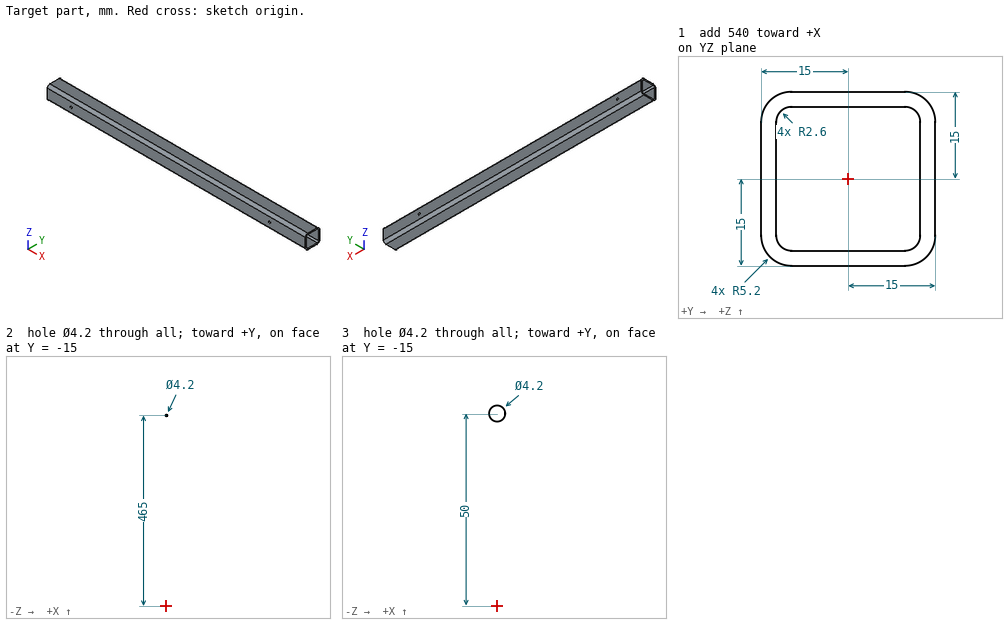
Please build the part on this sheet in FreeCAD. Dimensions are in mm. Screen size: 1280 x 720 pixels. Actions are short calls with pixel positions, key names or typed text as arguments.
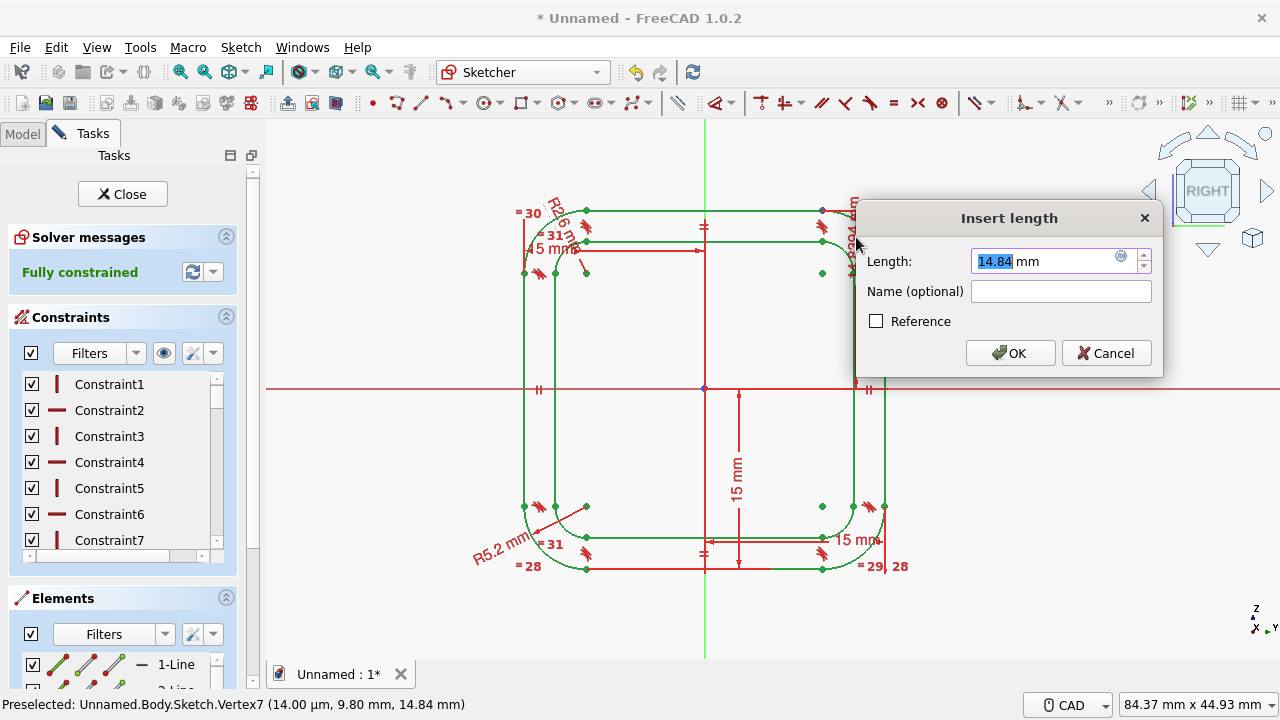
text(15)
key(Return)
key(Escape)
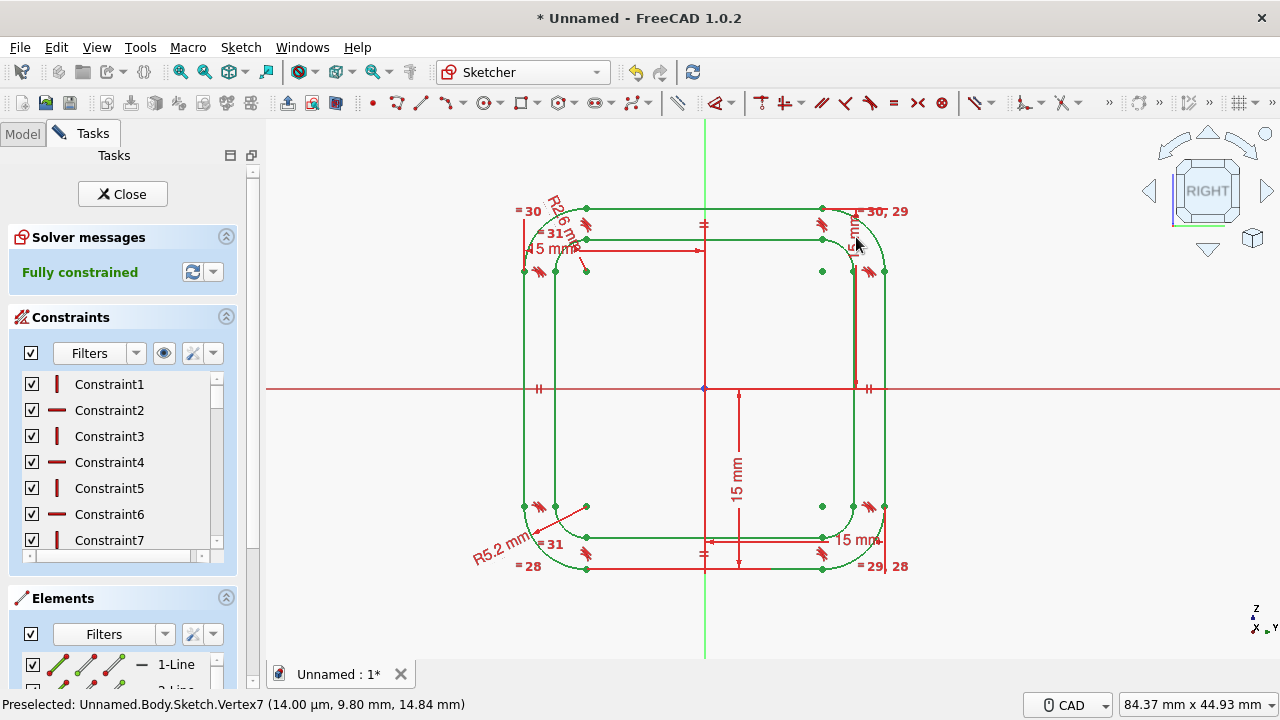
click(123, 194)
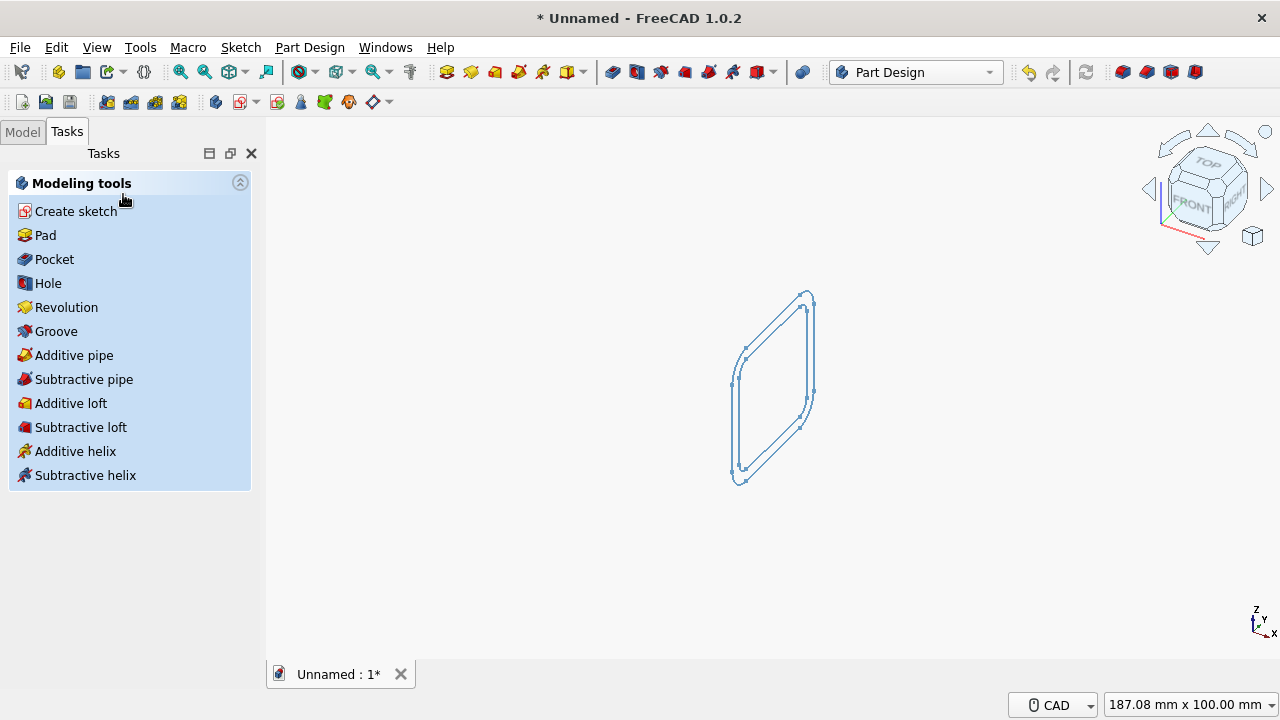
click(448, 72)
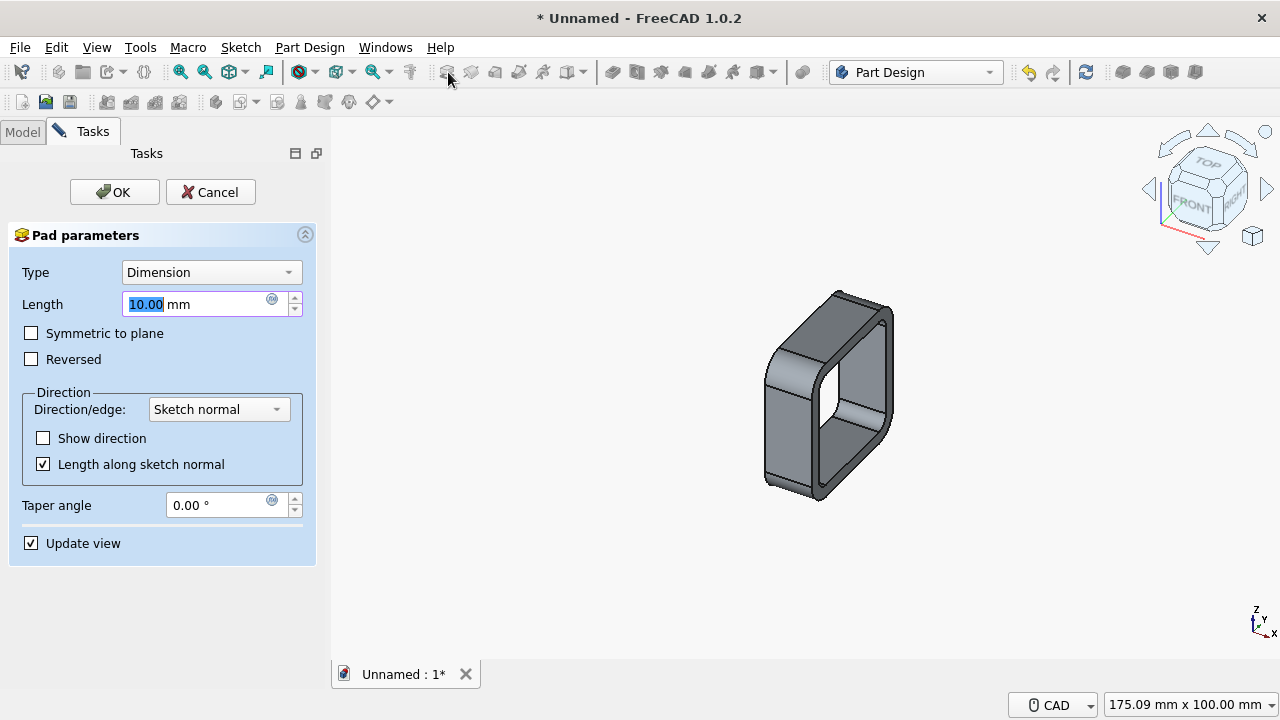
text(540)
key(Tab)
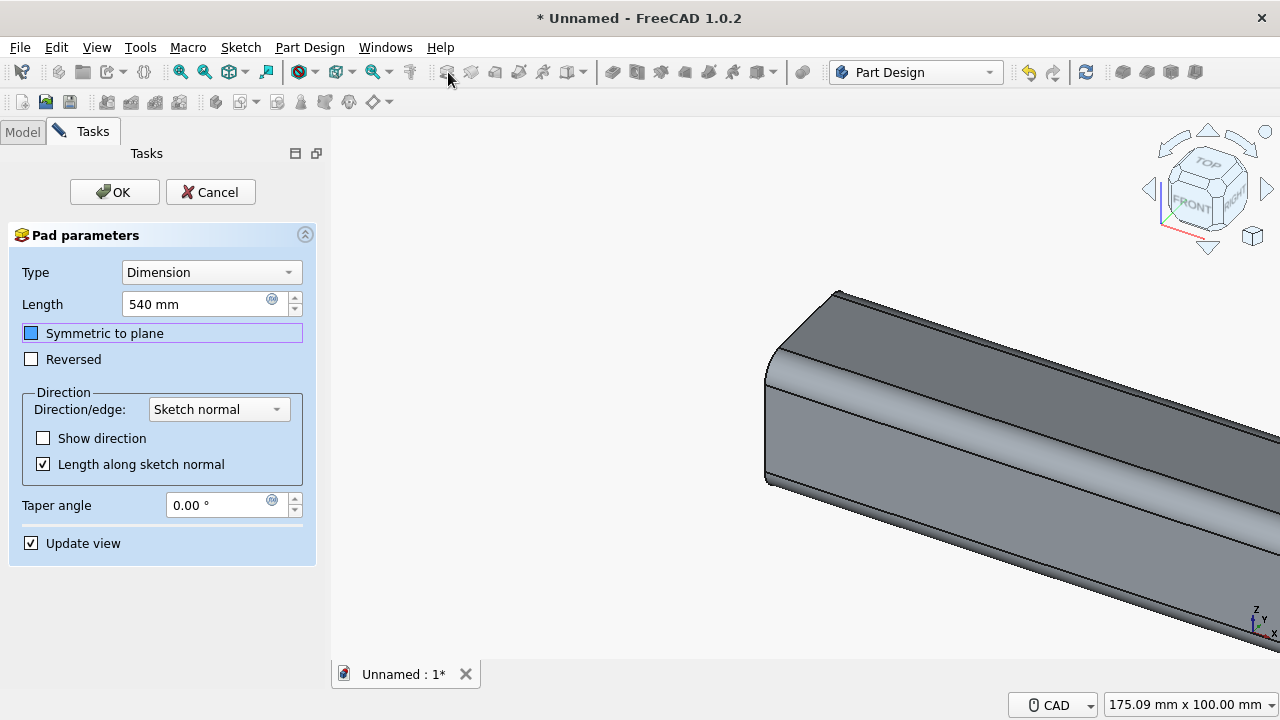
click(115, 192)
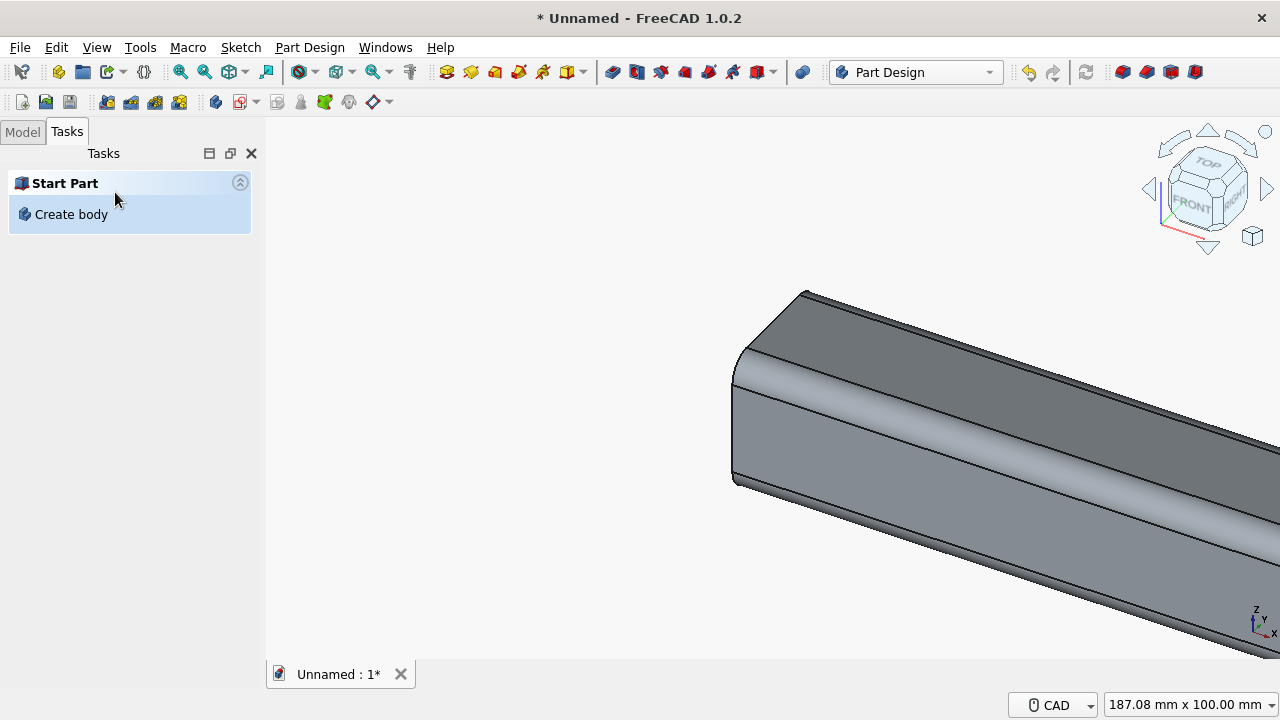
click(182, 72)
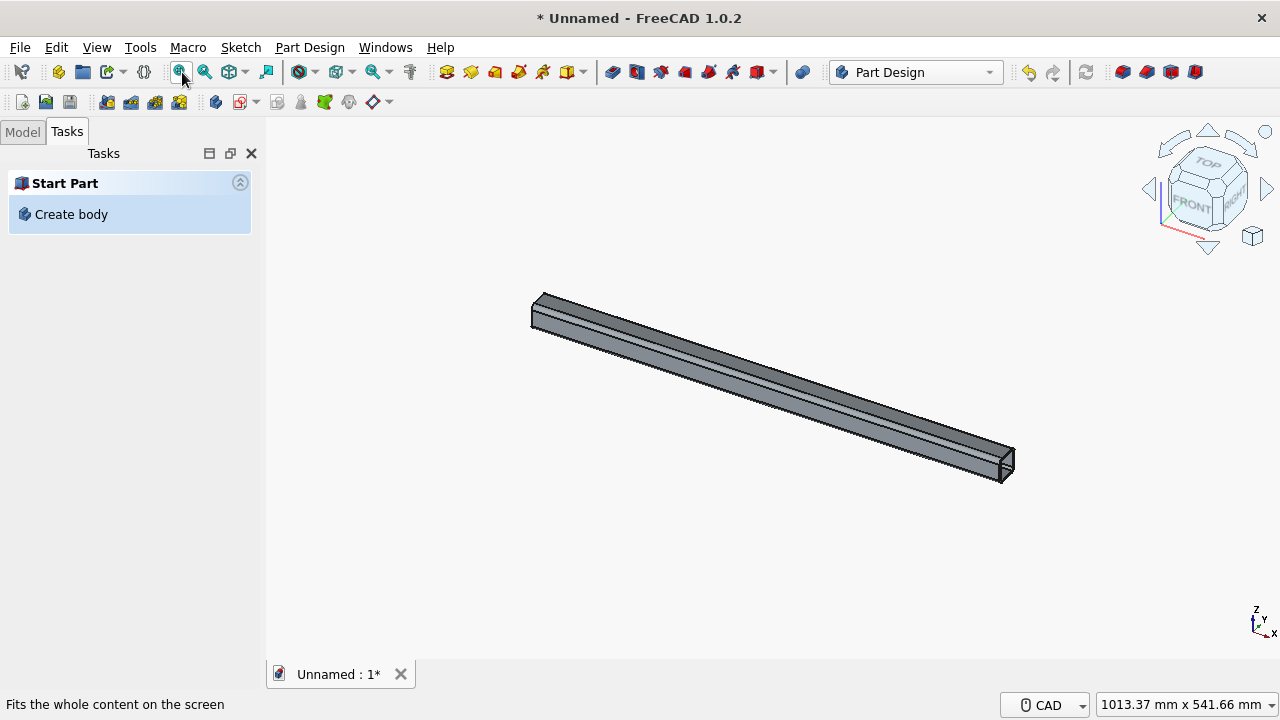
click(966, 463)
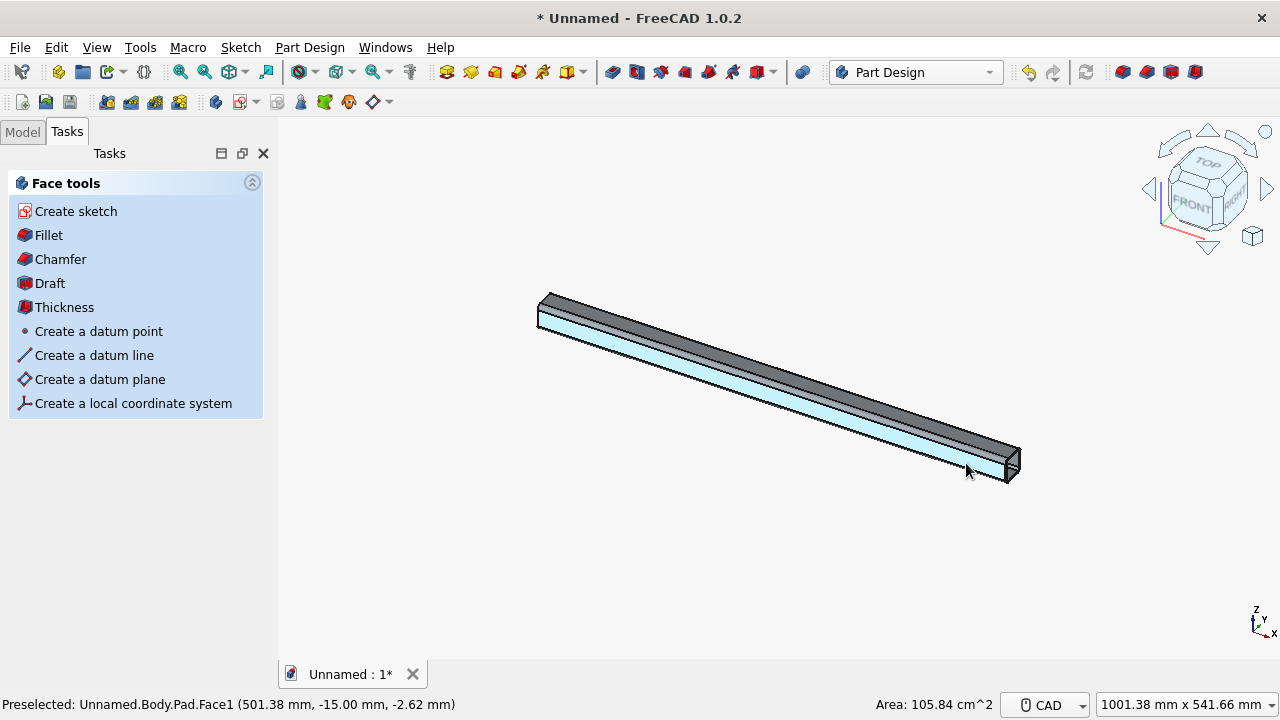
click(240, 102)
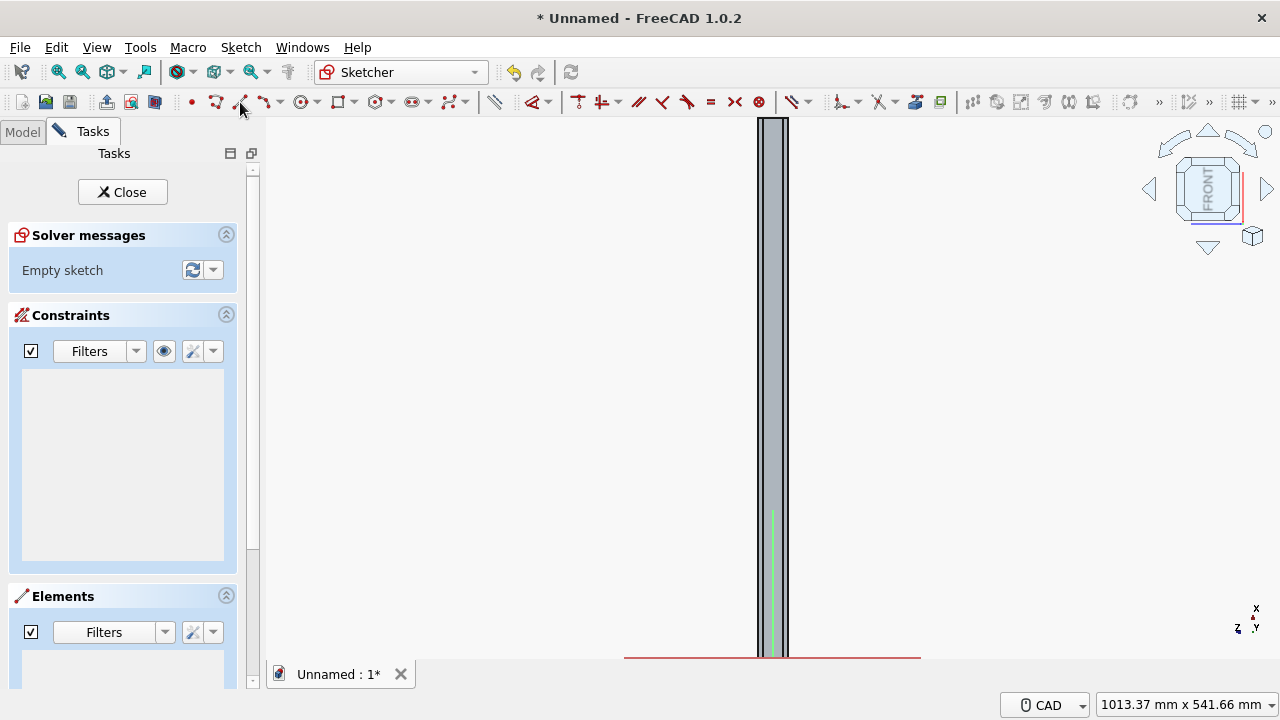
scroll(777, 183, up, 15)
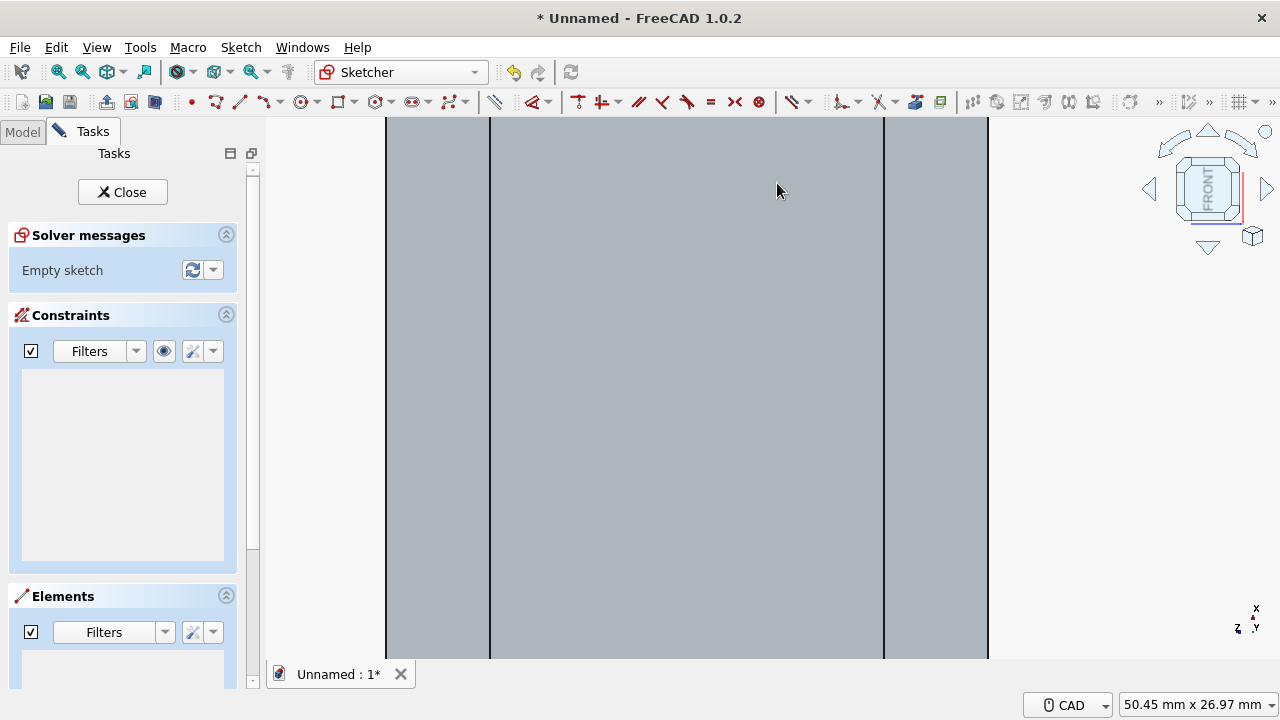
scroll(681, 376, up, 7)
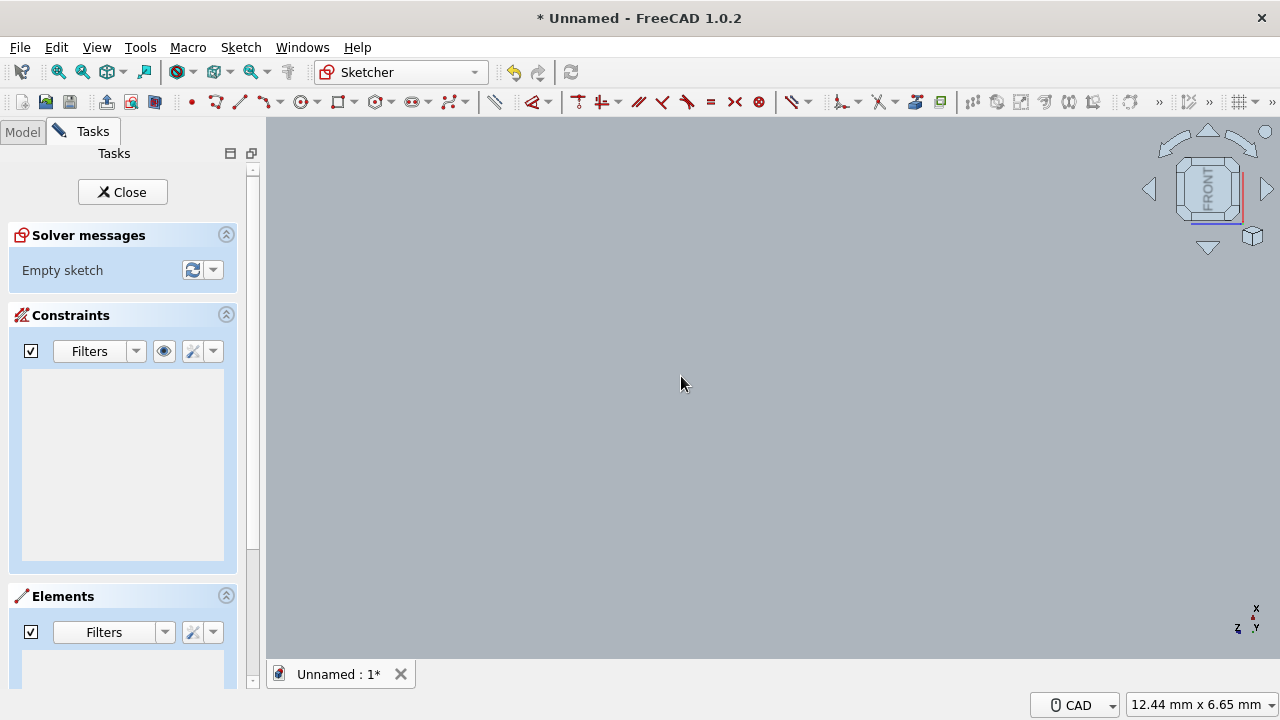
click(302, 102)